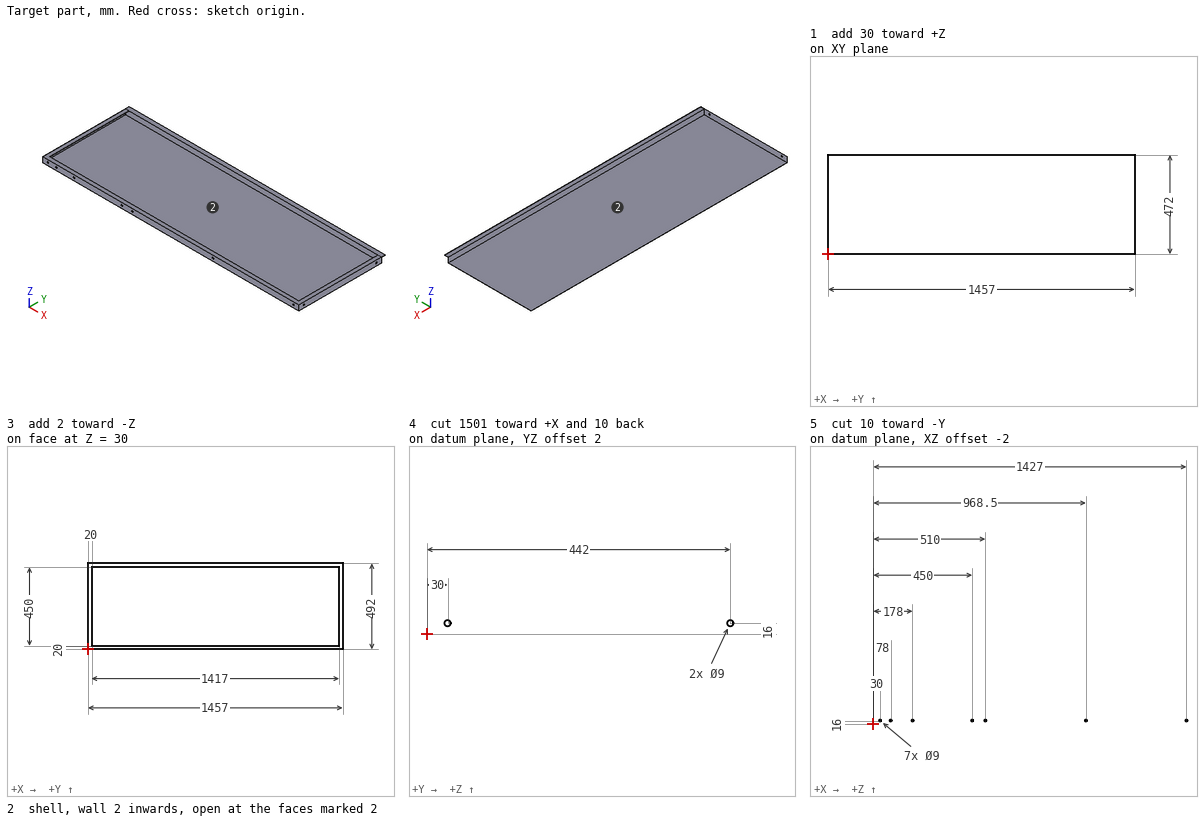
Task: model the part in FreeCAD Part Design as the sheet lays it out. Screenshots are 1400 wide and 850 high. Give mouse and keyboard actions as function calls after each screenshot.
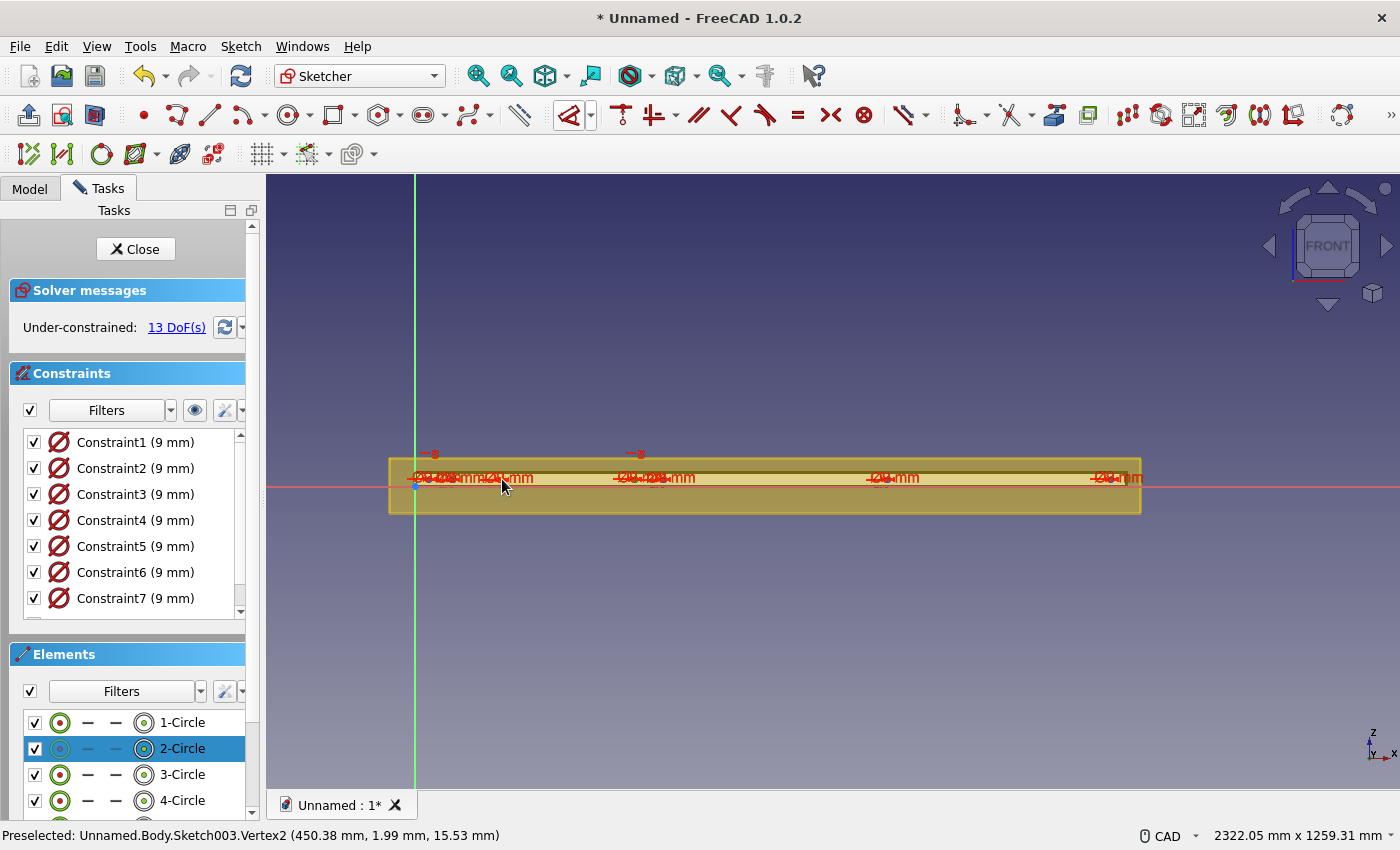
click(1112, 479)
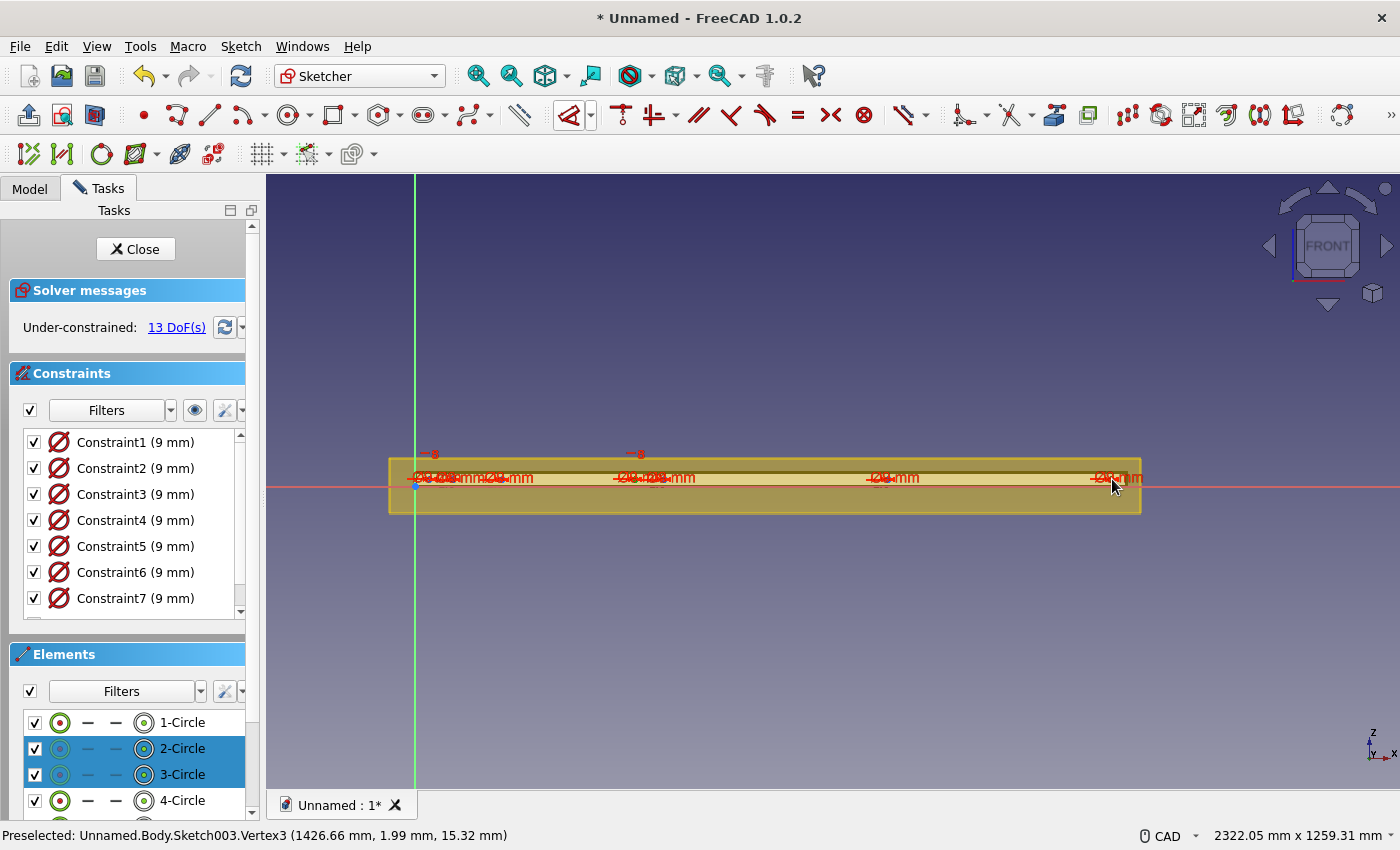
key(h)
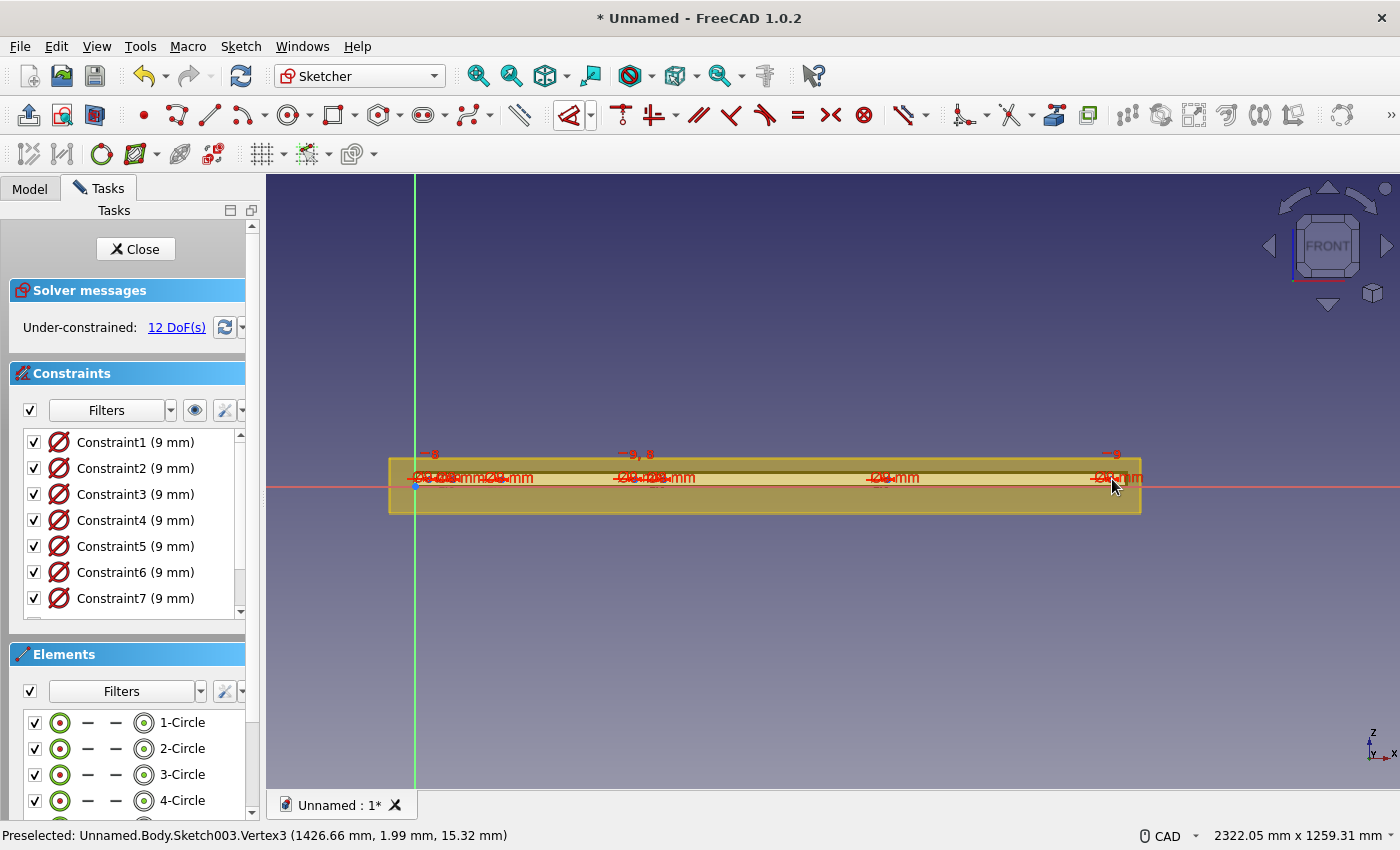
click(1112, 479)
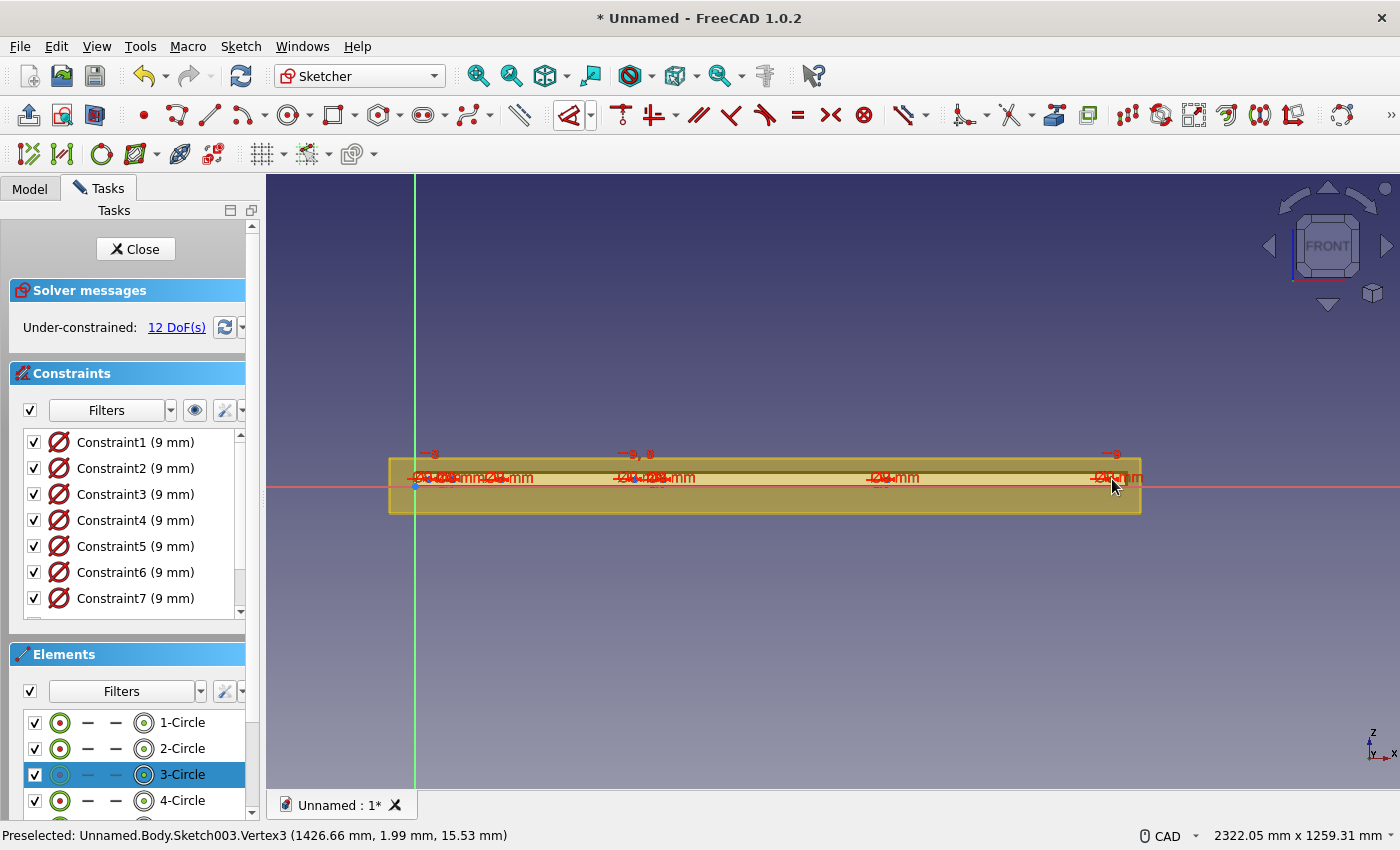
click(888, 480)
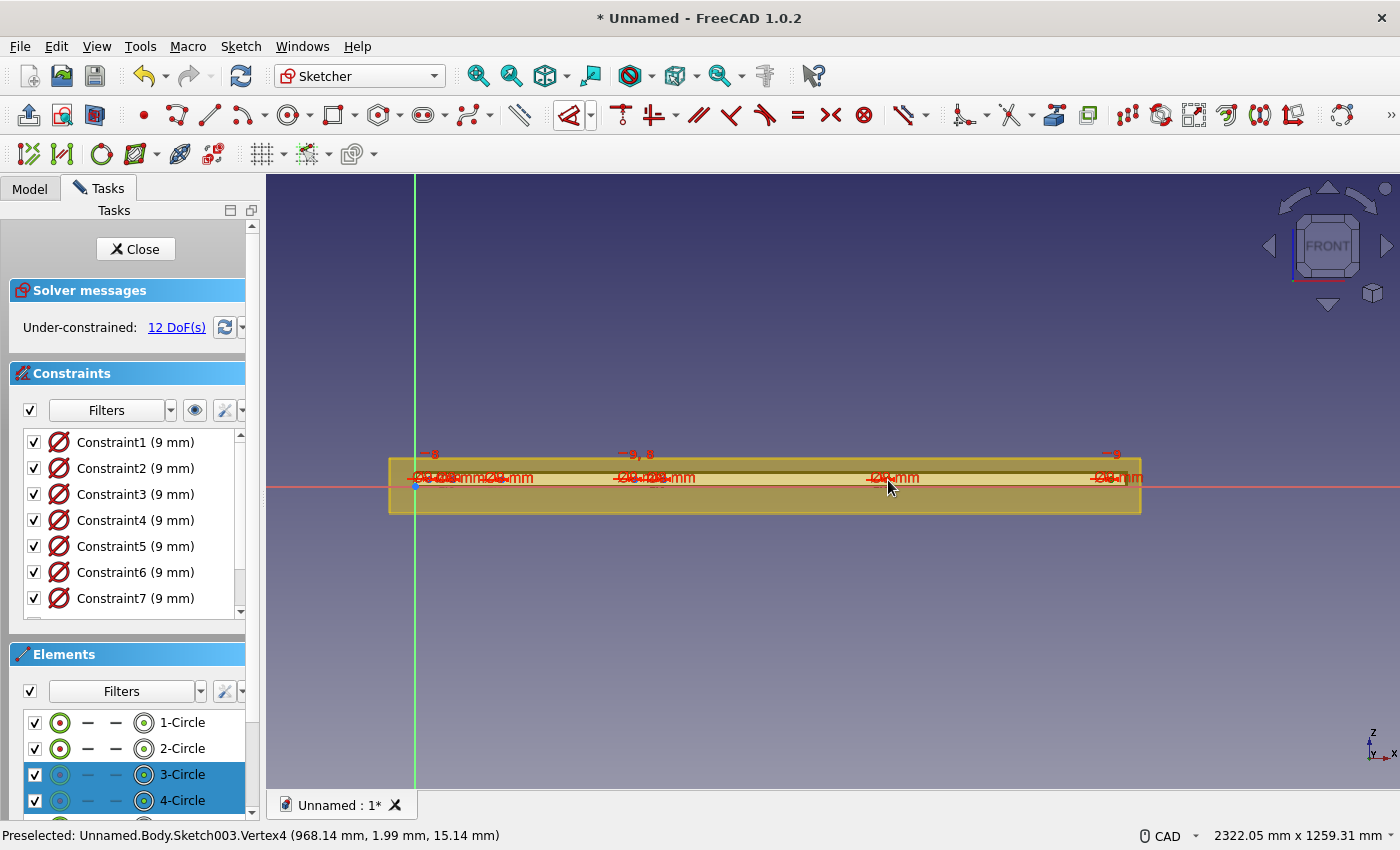
click(676, 116)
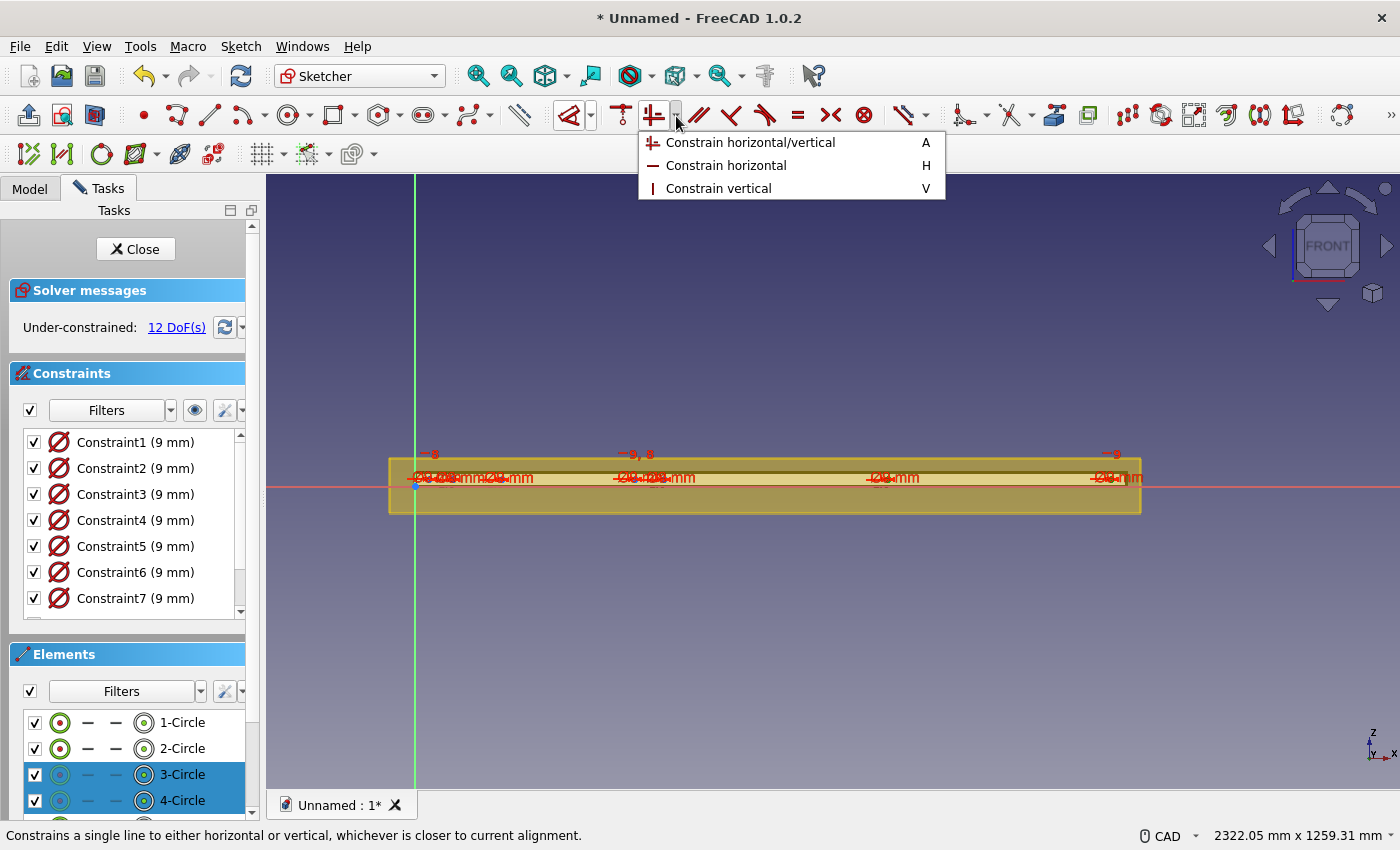
click(792, 166)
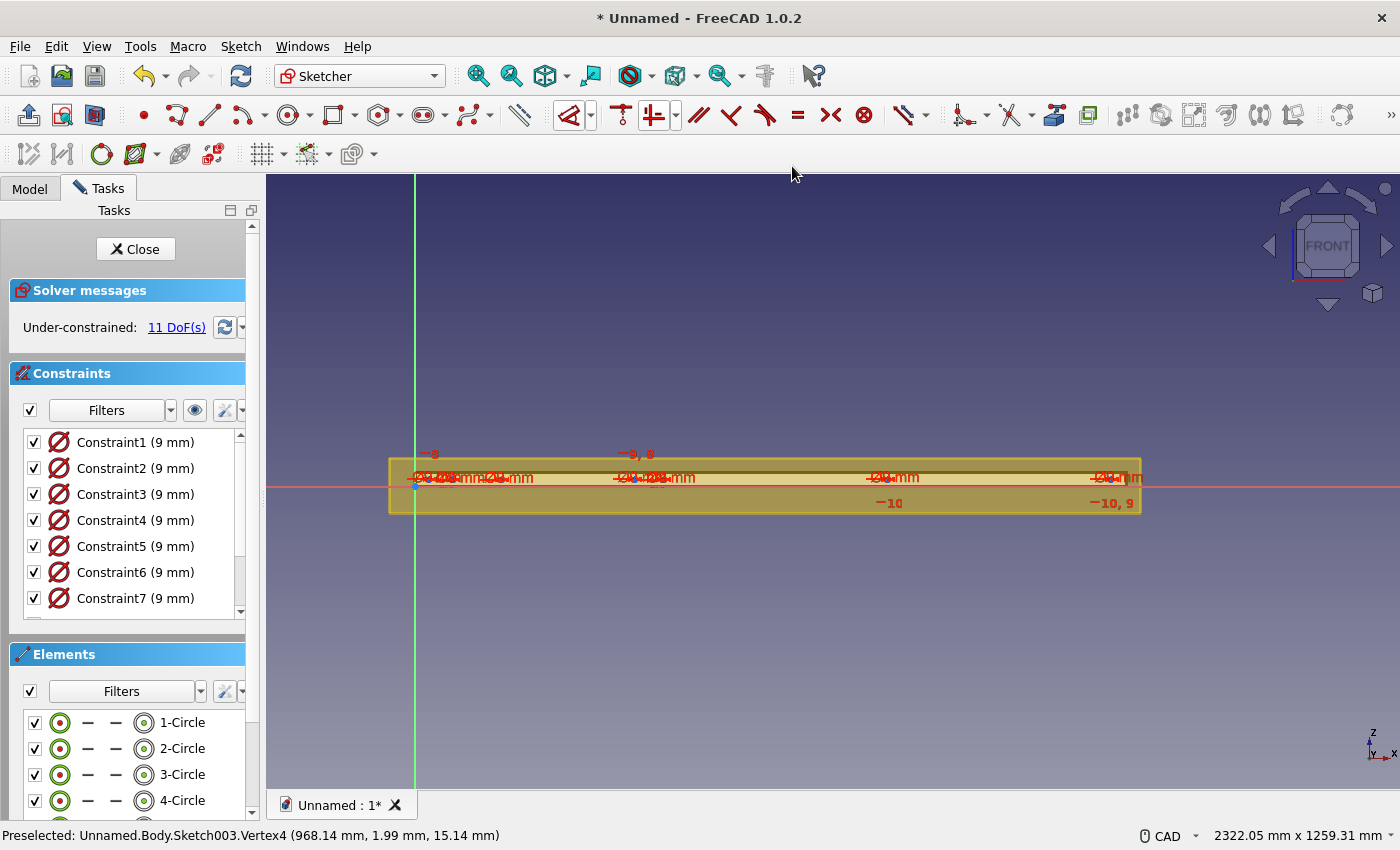
click(635, 479)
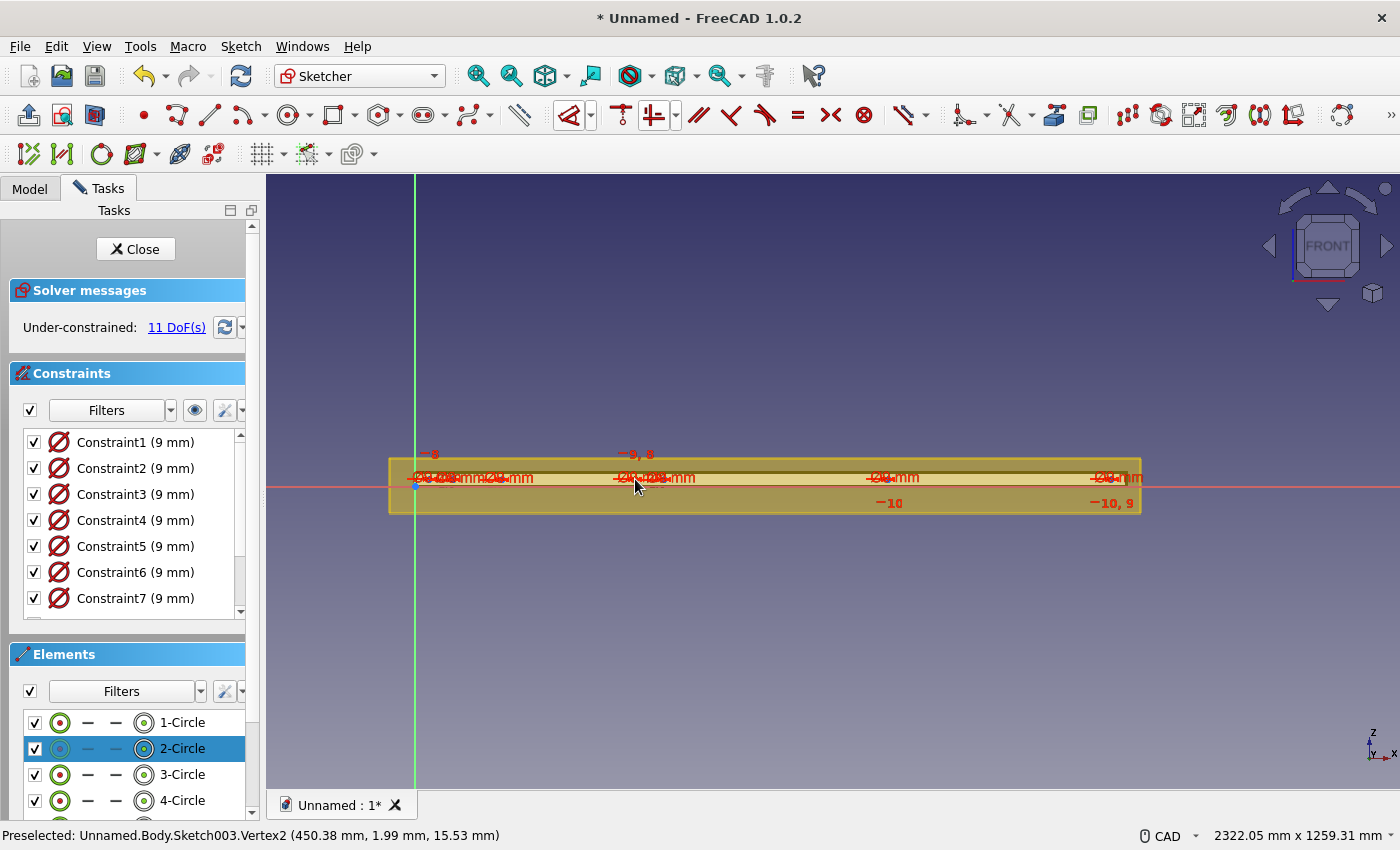
click(664, 480)